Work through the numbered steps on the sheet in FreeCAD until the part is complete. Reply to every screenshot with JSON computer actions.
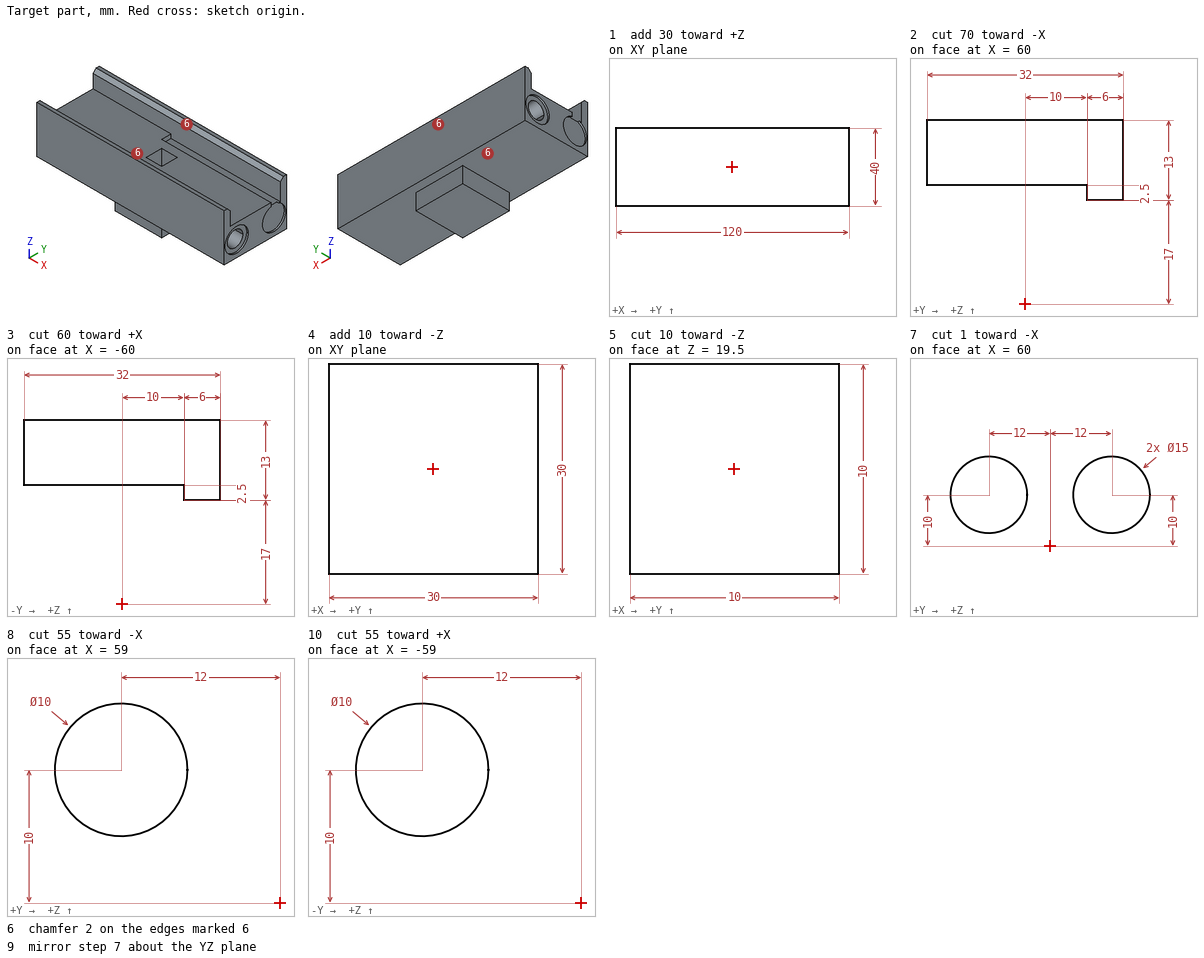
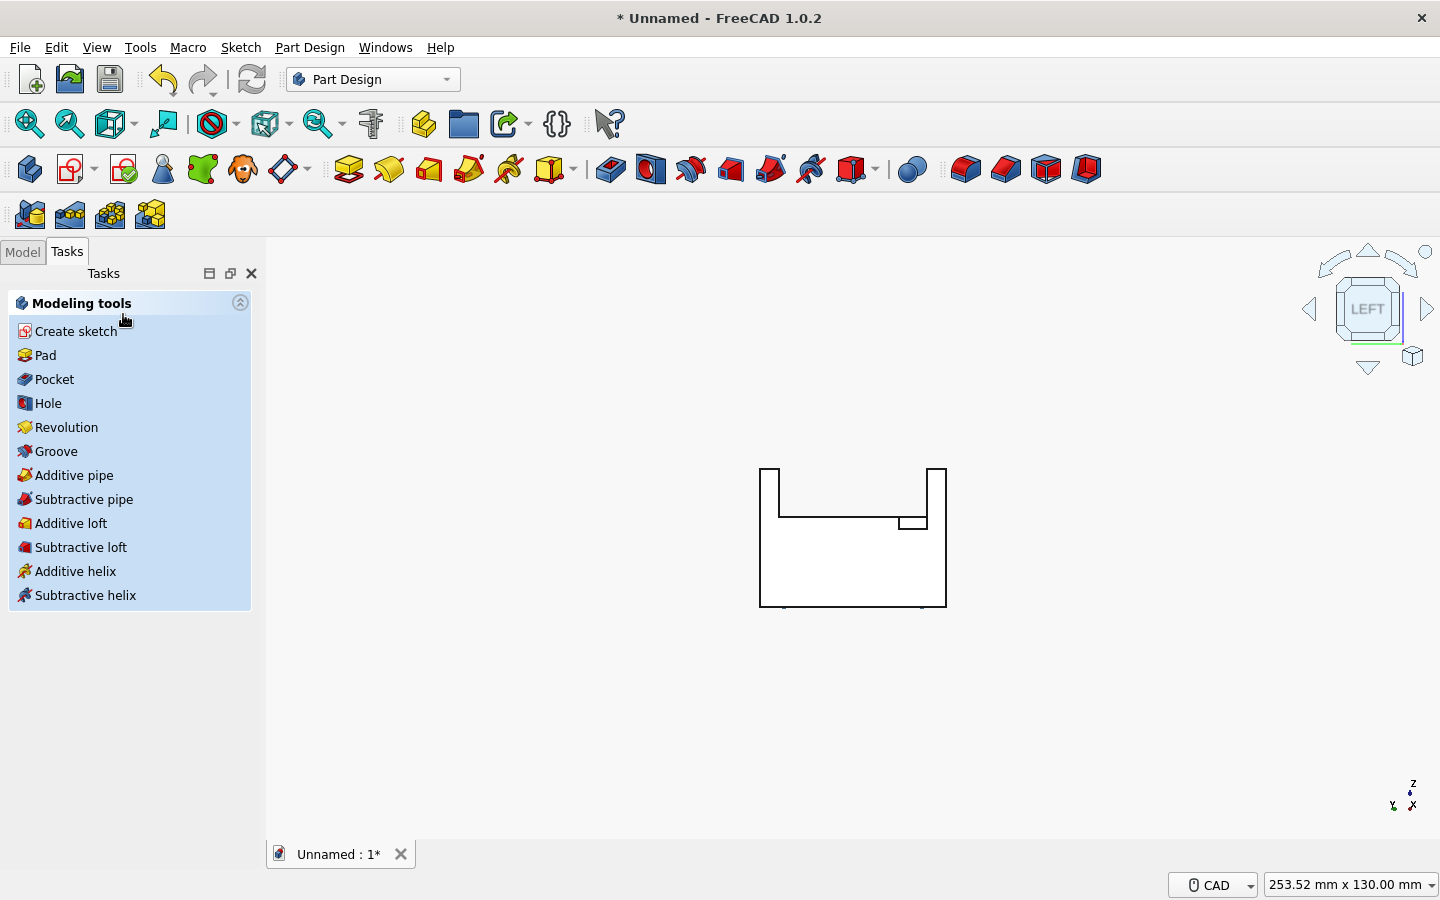
{"action": "left_click", "coordinate": [350, 170]}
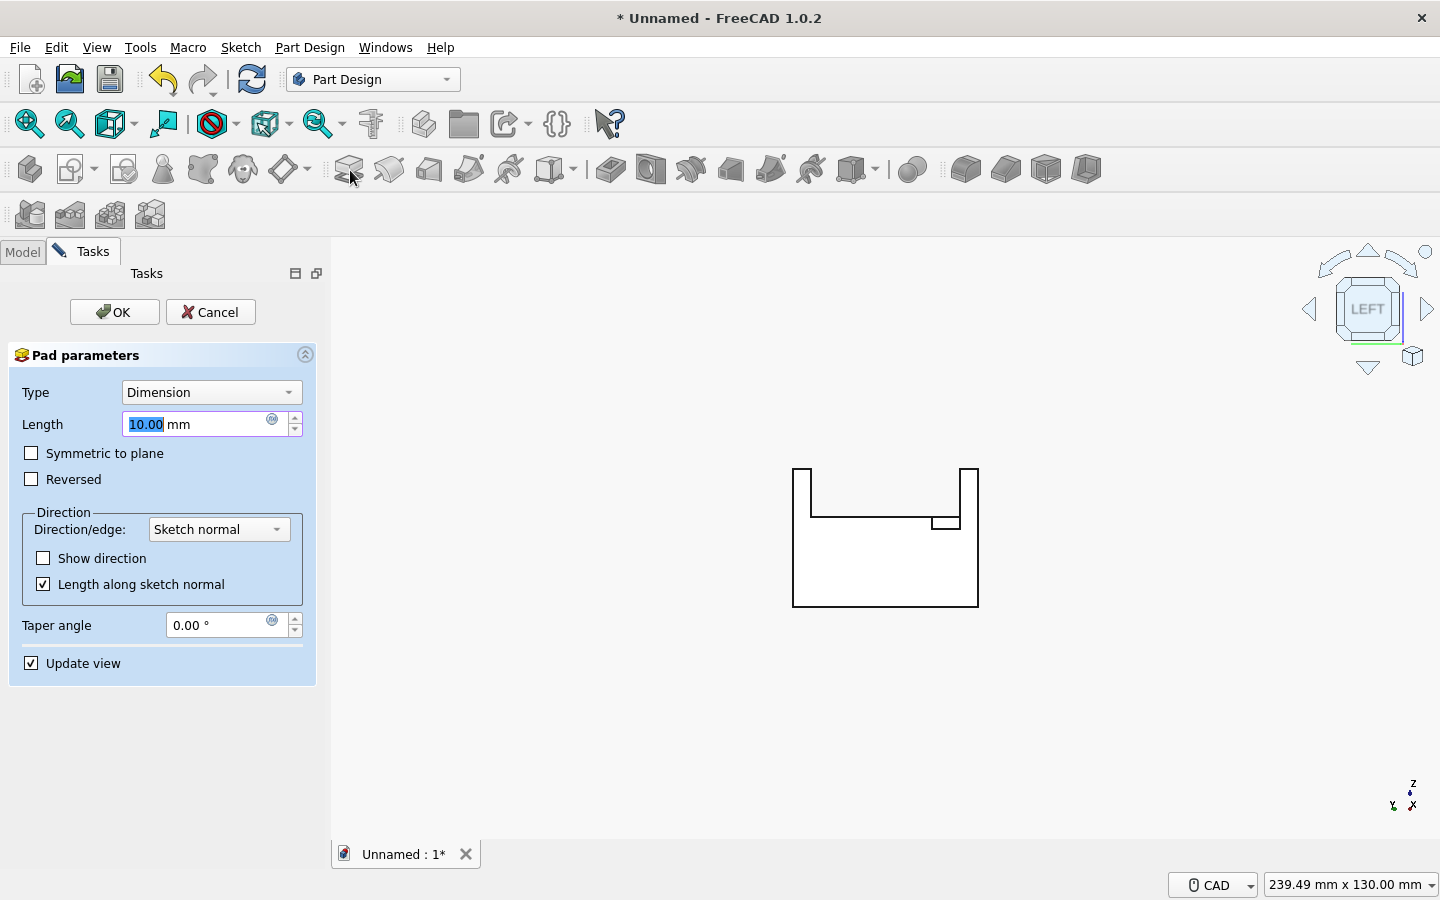
{"action": "type", "text": "10"}
{"action": "key", "text": "Tab"}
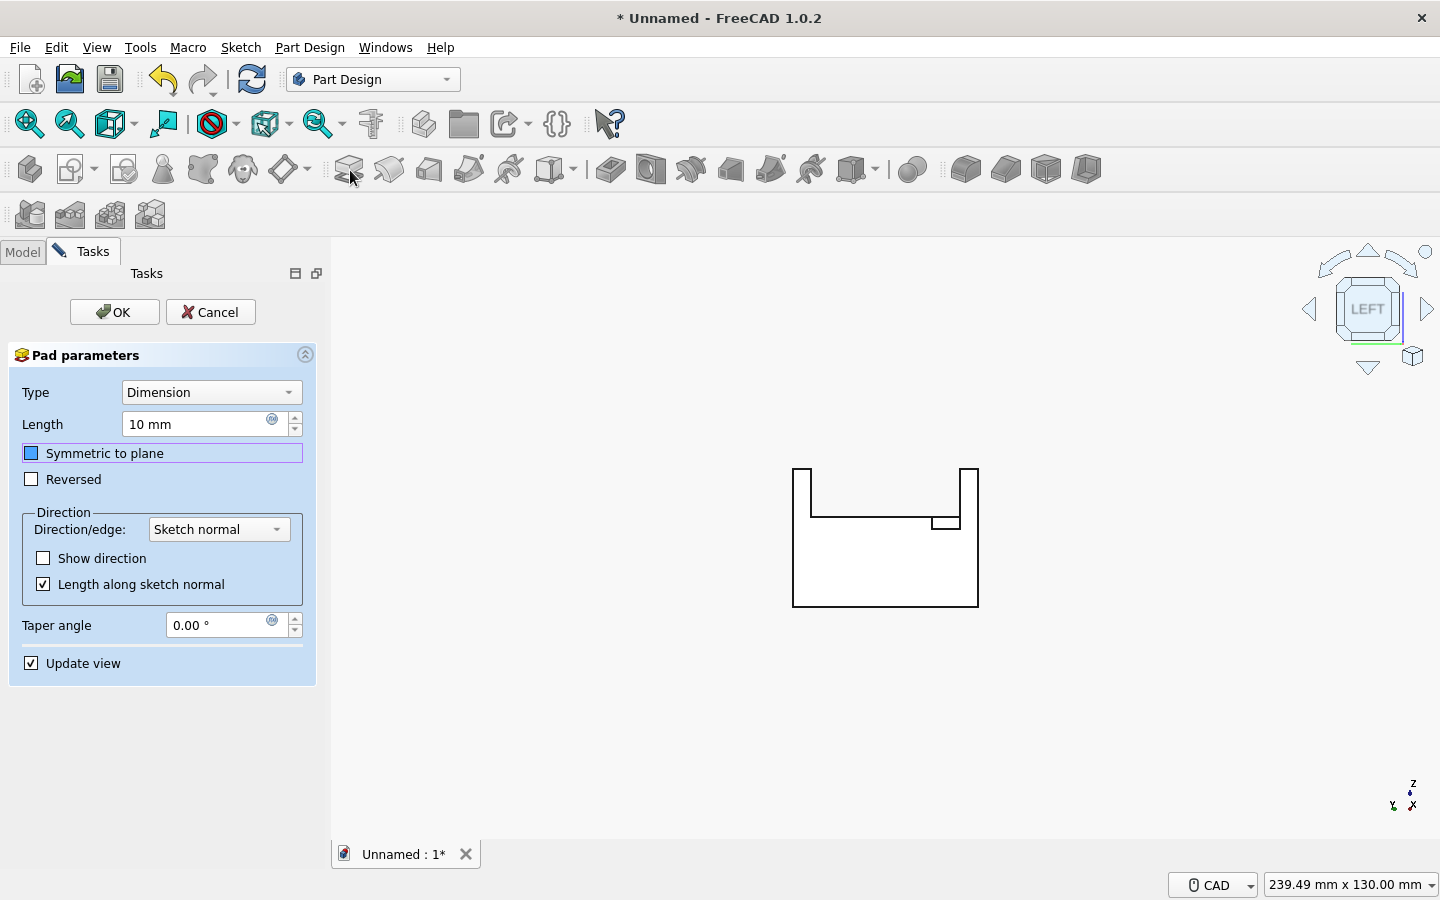
{"action": "left_click", "coordinate": [30, 479]}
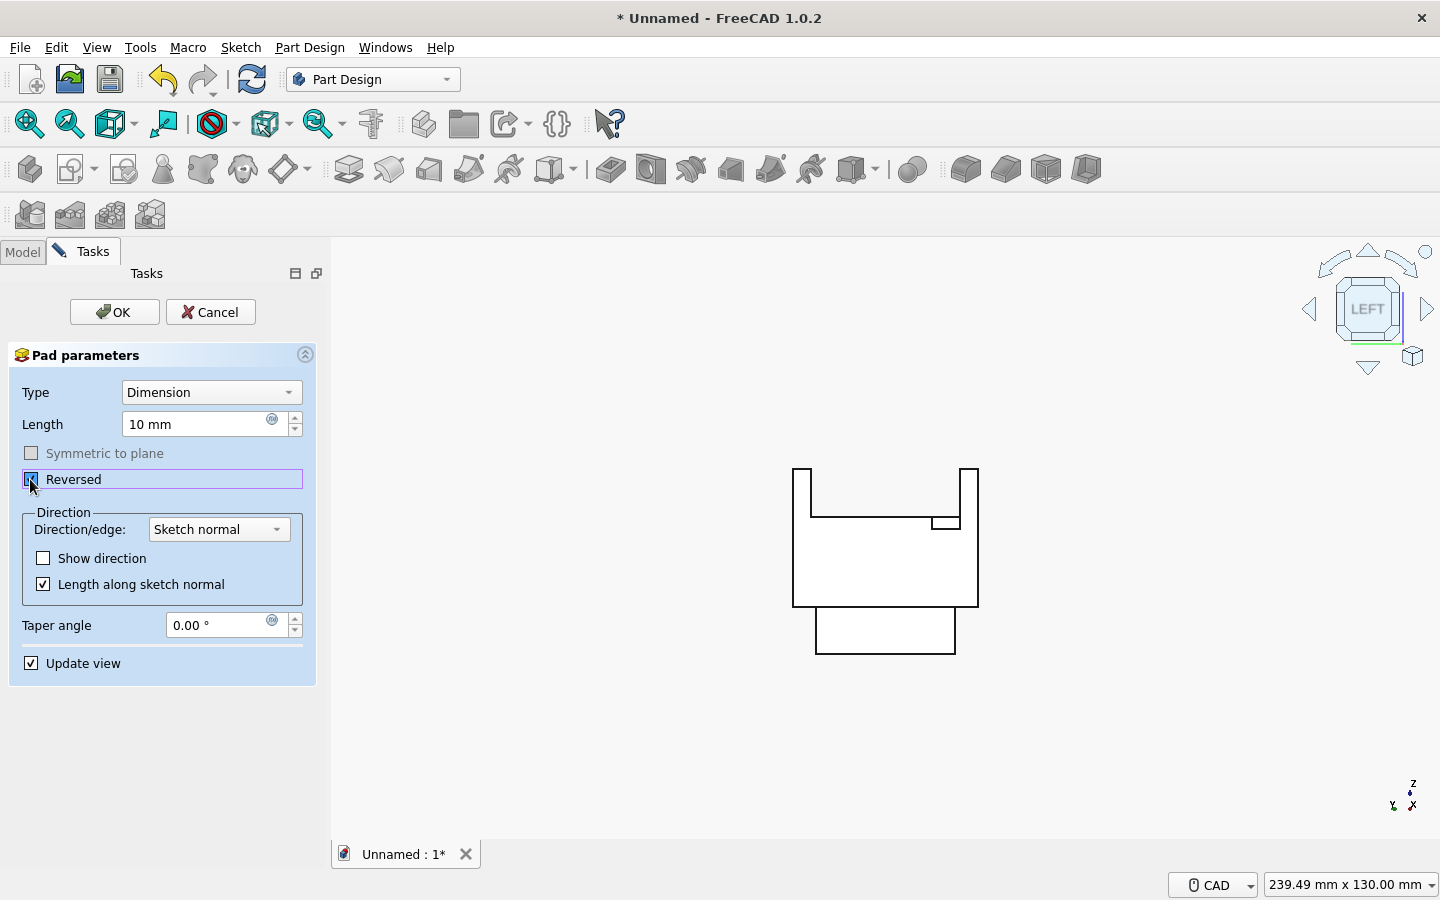
{"action": "left_click", "coordinate": [115, 312]}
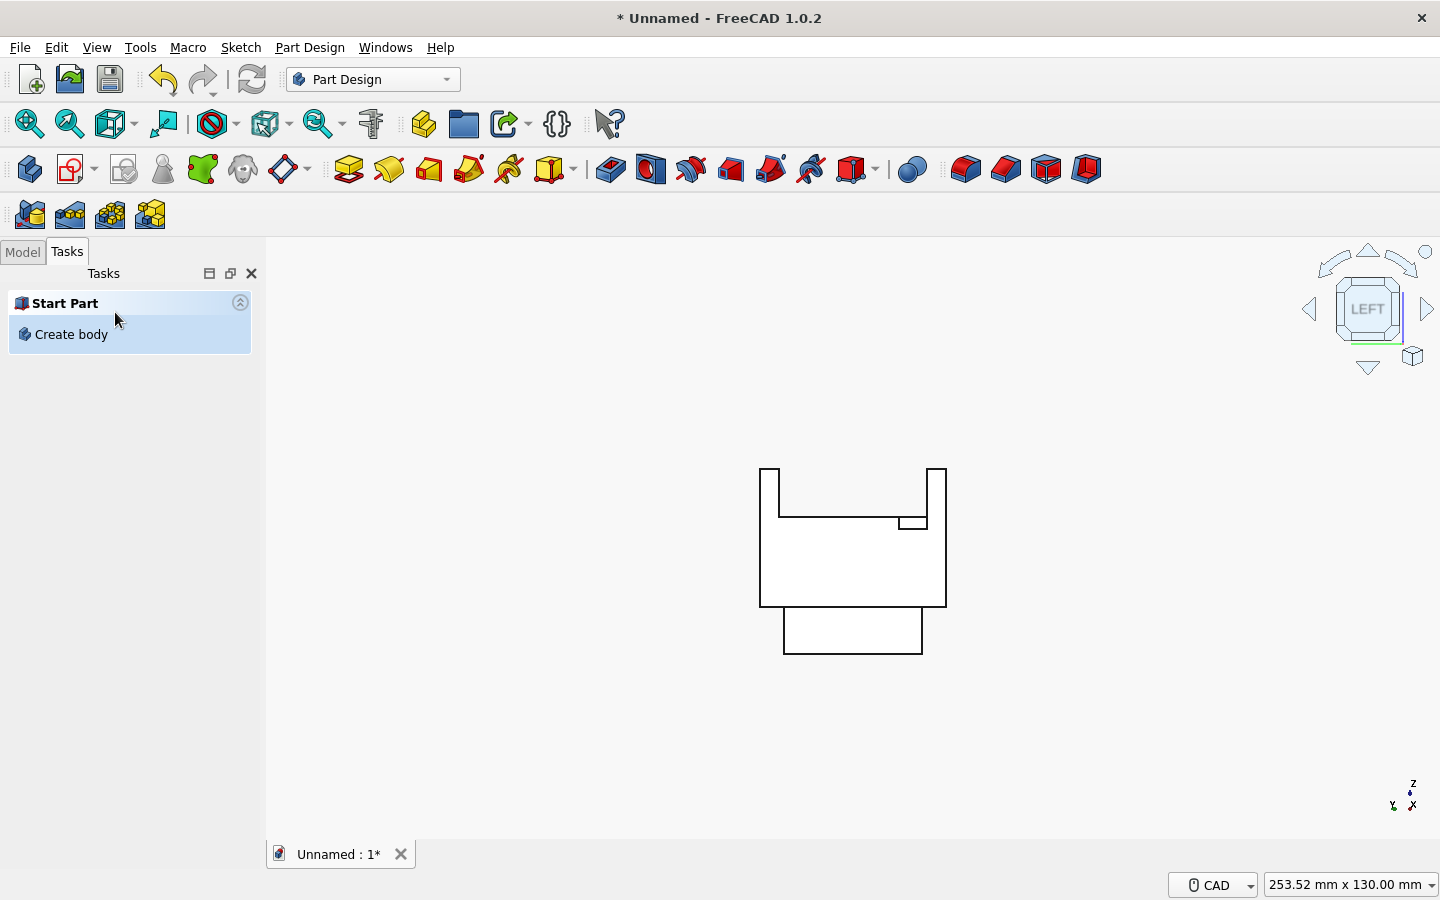
{"action": "key", "text": "v f"}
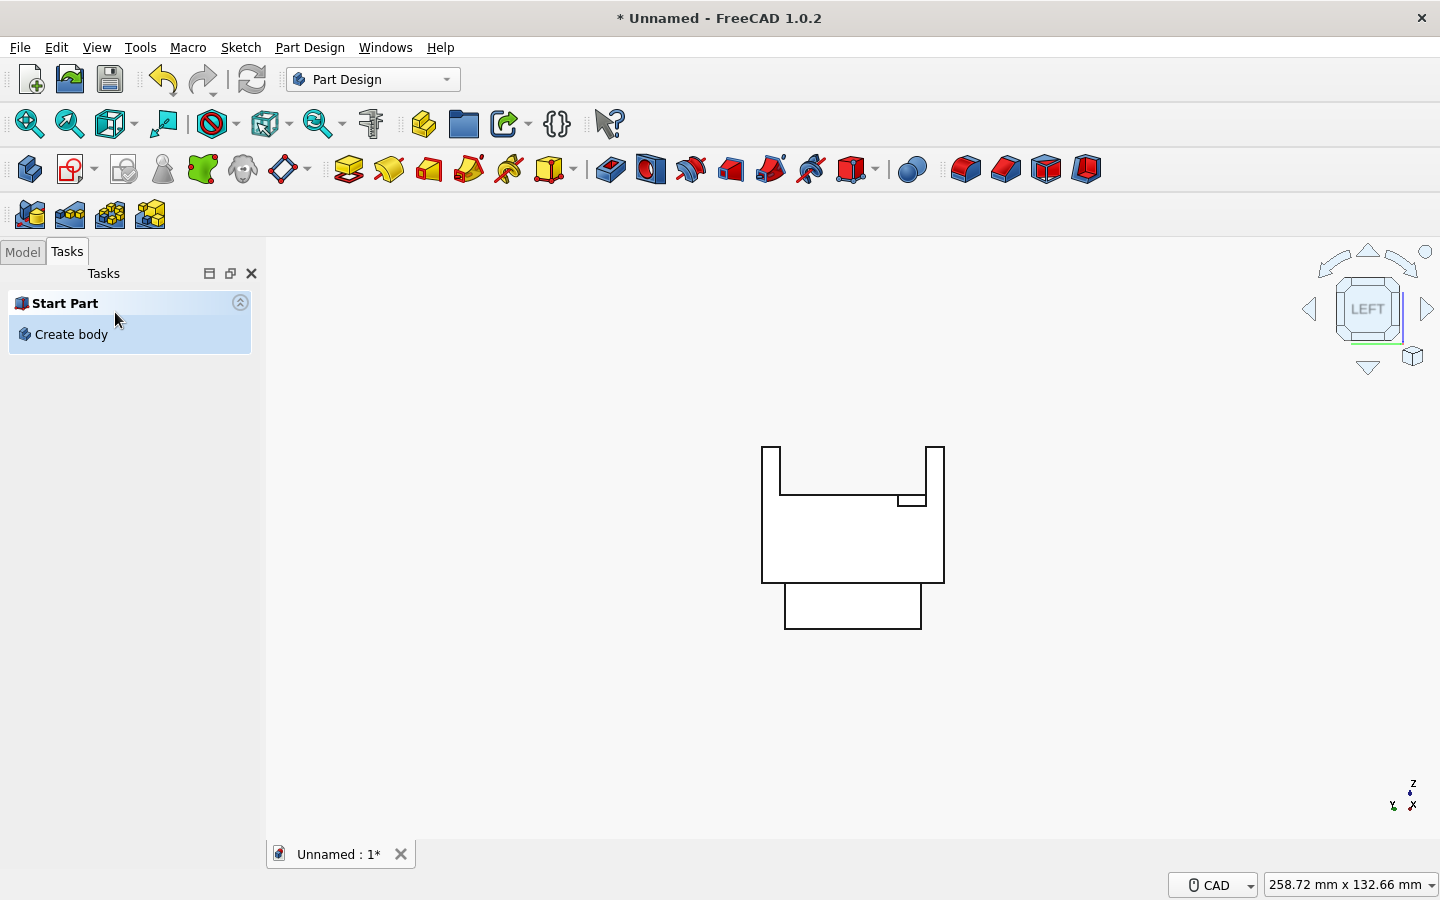
{"action": "key", "text": "0"}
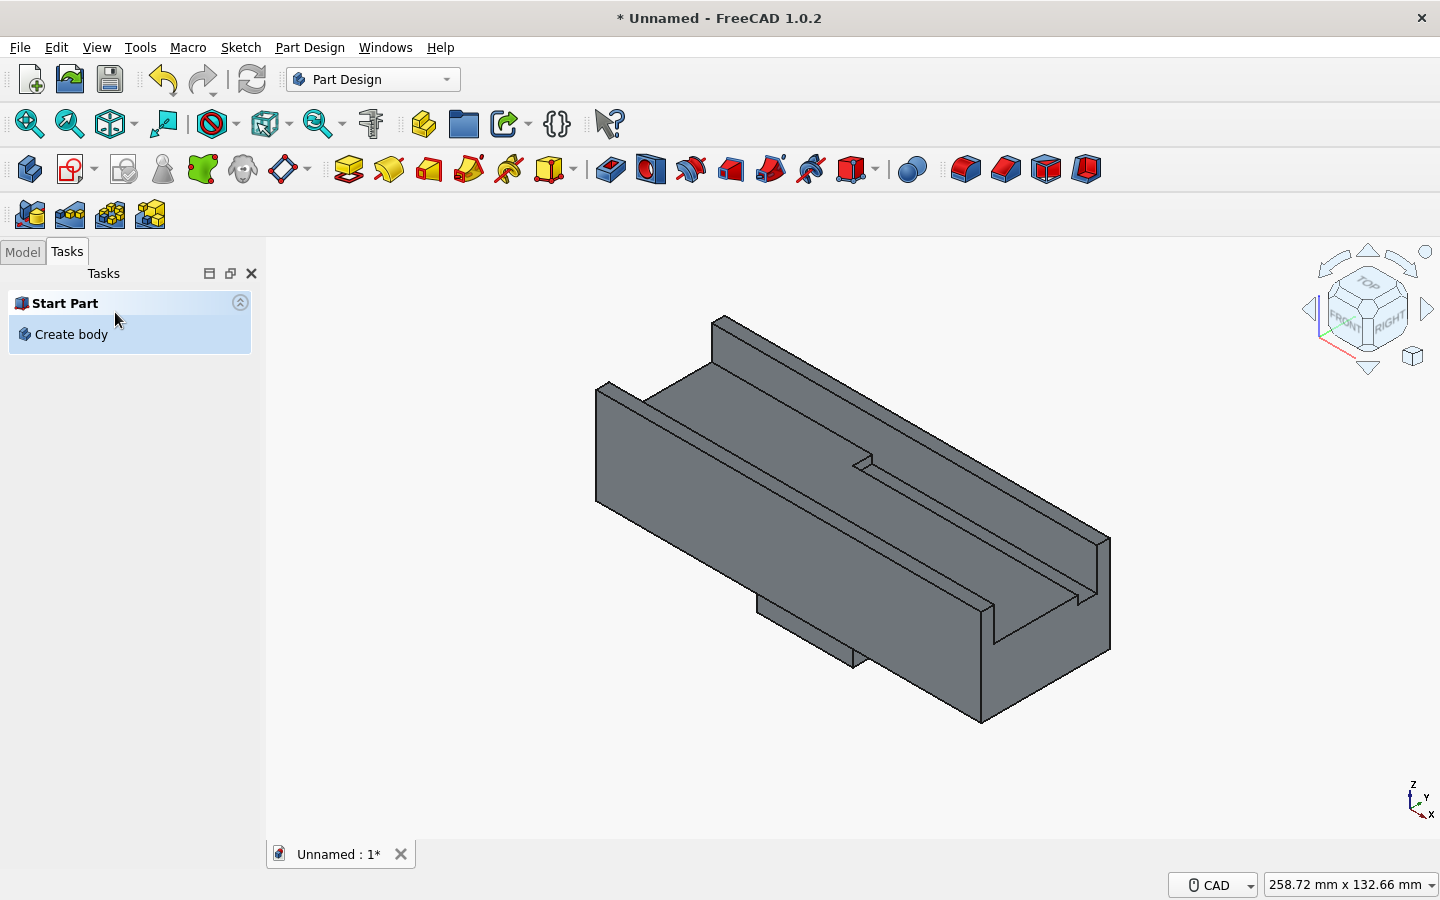
{"action": "left_click", "coordinate": [758, 430]}